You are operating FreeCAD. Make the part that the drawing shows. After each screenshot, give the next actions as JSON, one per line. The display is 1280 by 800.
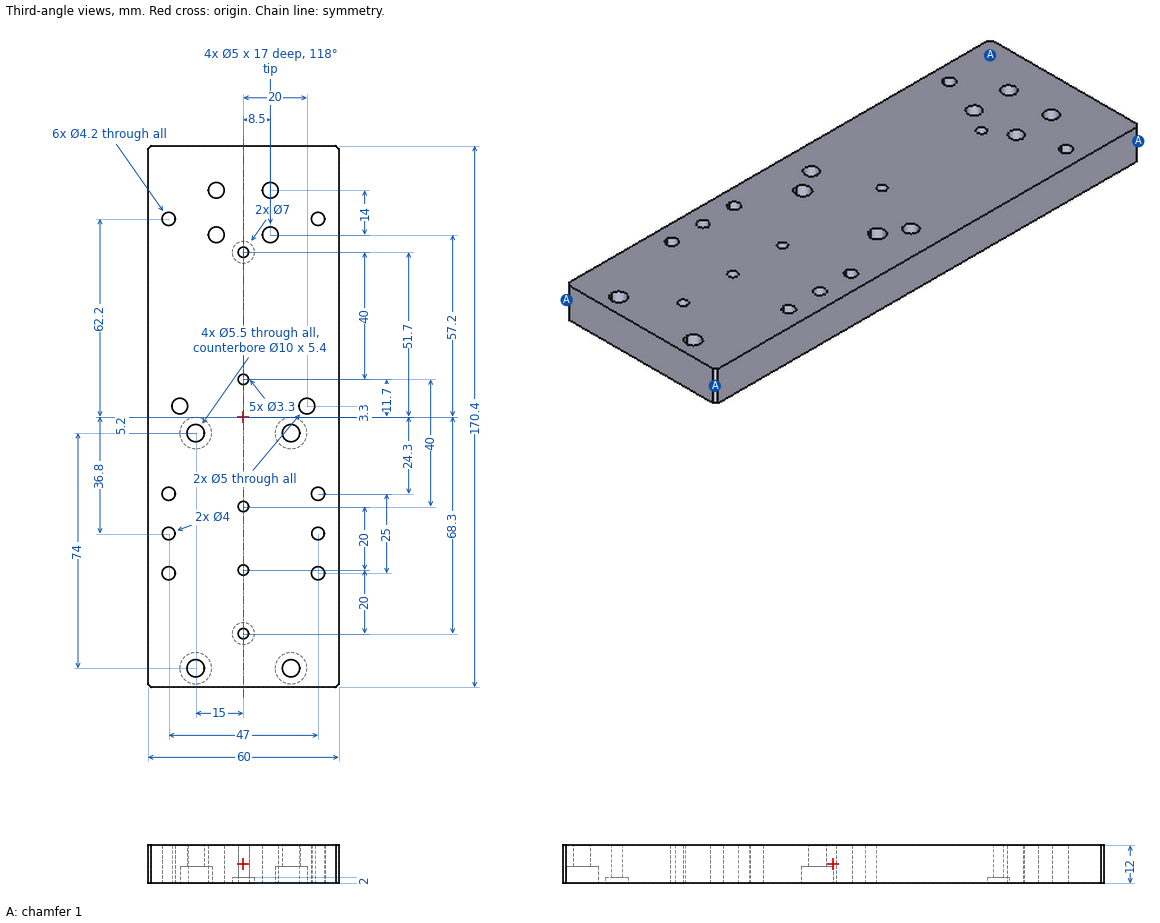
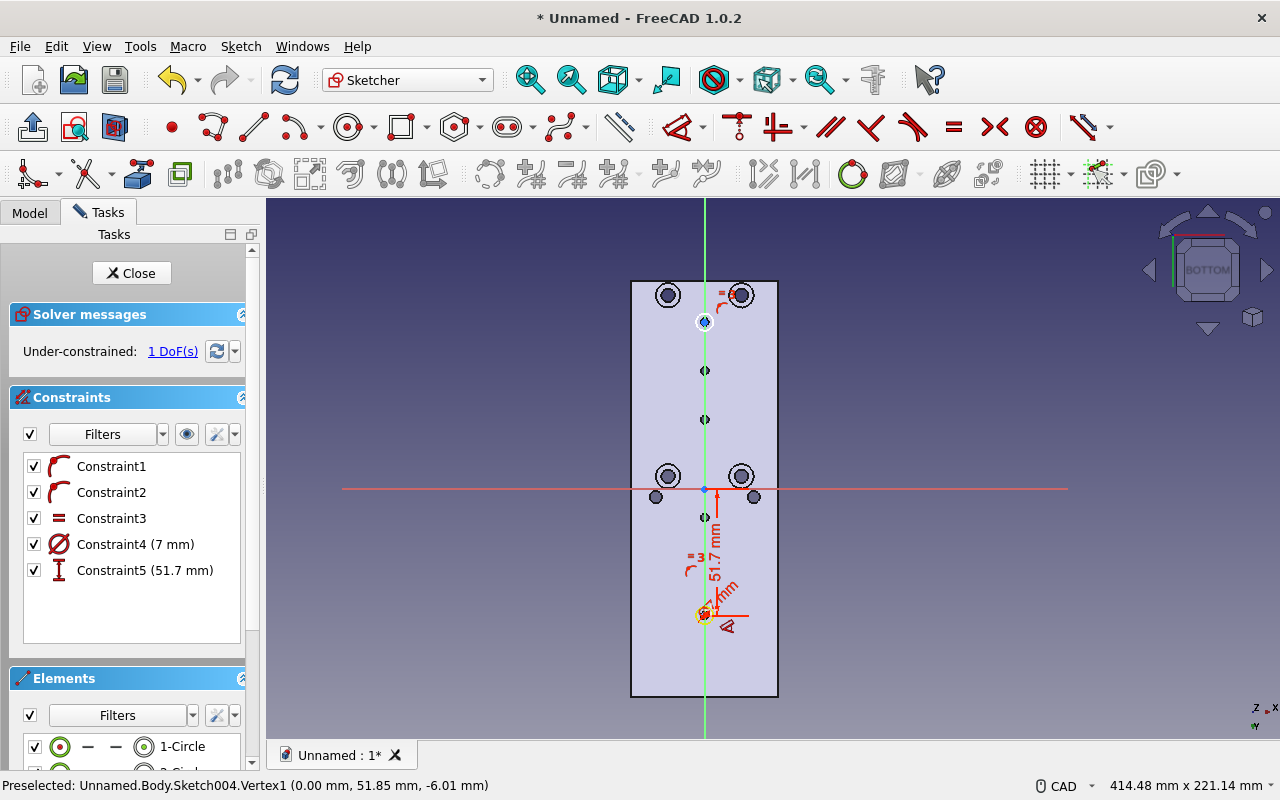
{"action": "left_click", "coordinate": [705, 322]}
{"action": "left_click", "coordinate": [739, 406]}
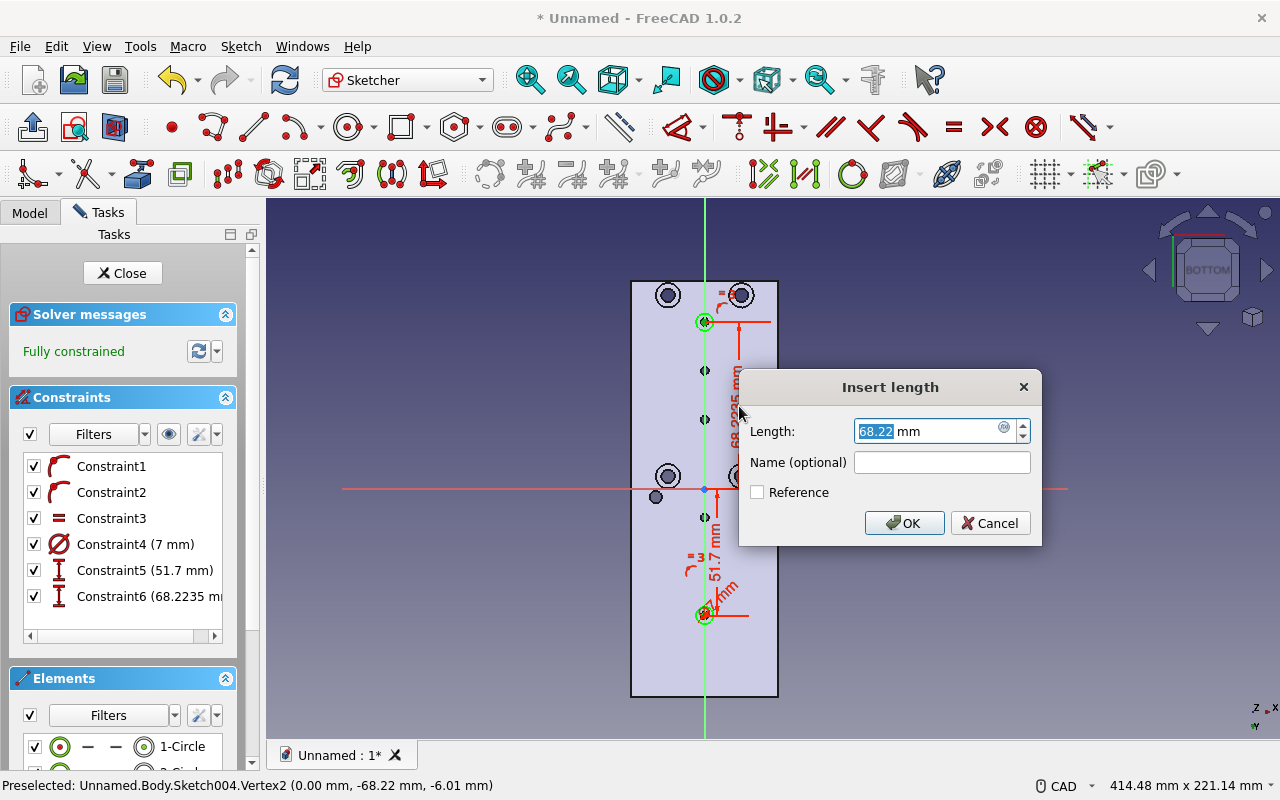
{"action": "type", "text": "68.3"}
{"action": "key", "text": "Return"}
{"action": "key", "text": "Escape"}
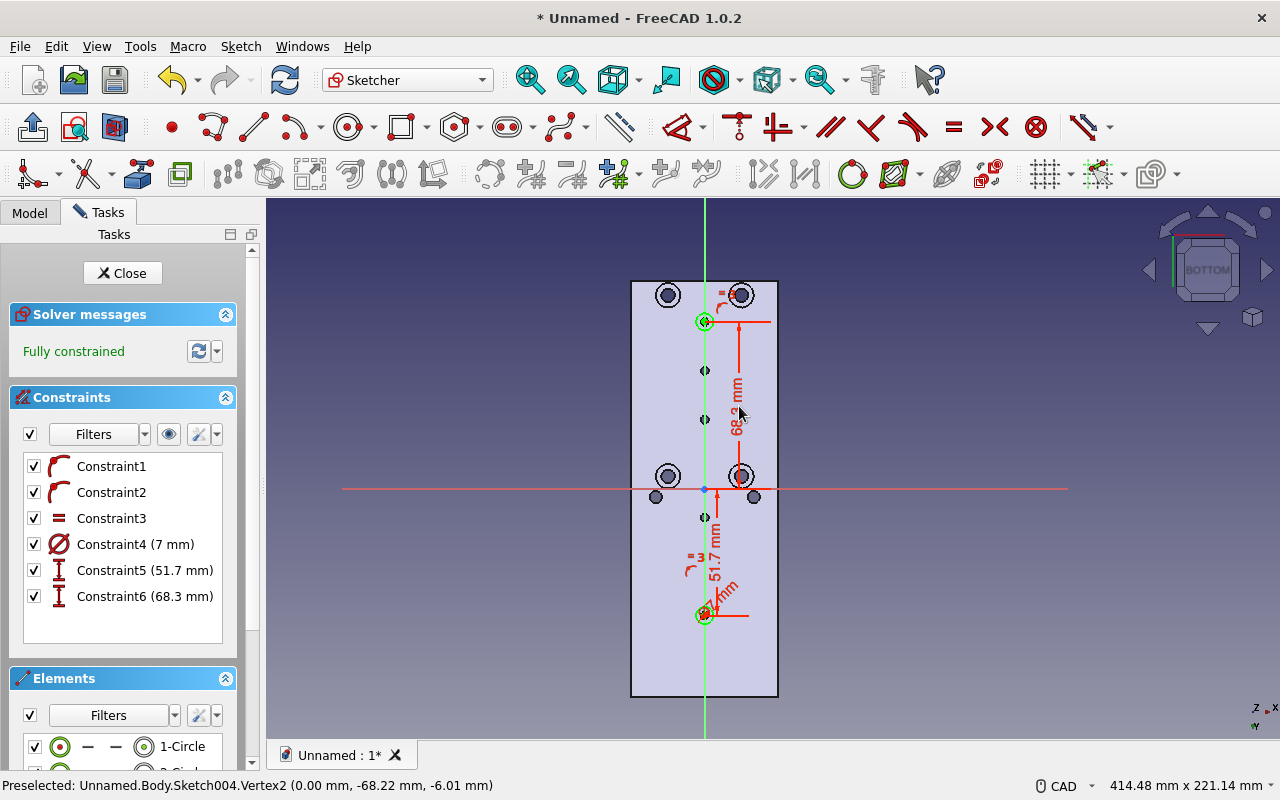
{"action": "left_click", "coordinate": [123, 273]}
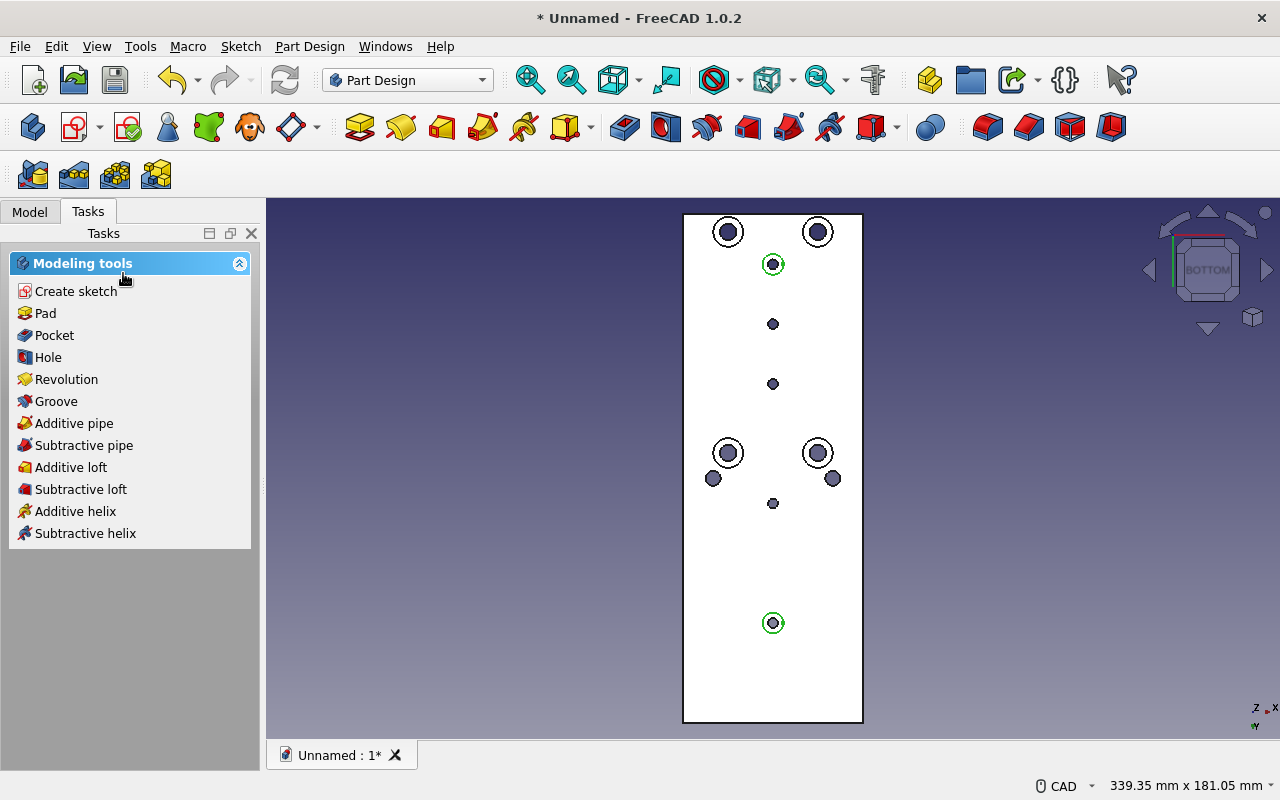
{"action": "left_click", "coordinate": [625, 128]}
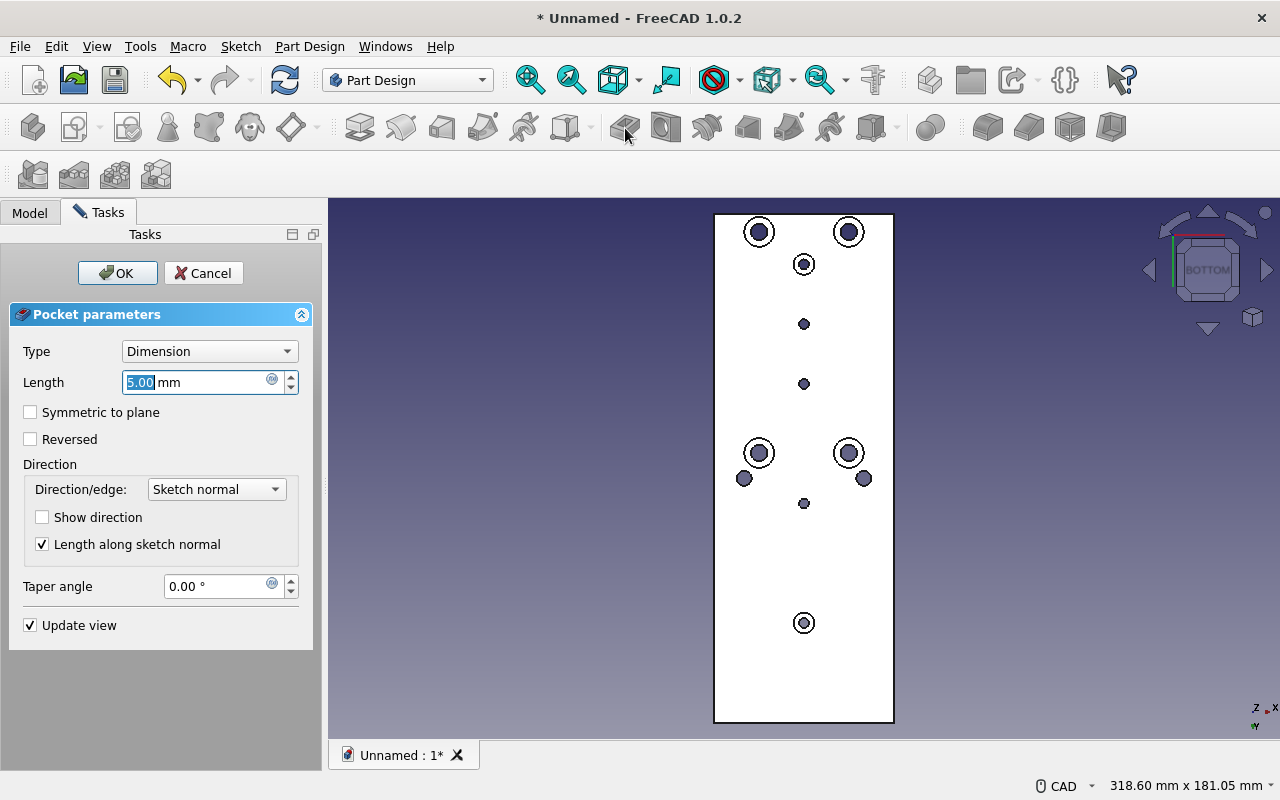
{"action": "type", "text": "2"}
{"action": "key", "text": "Tab"}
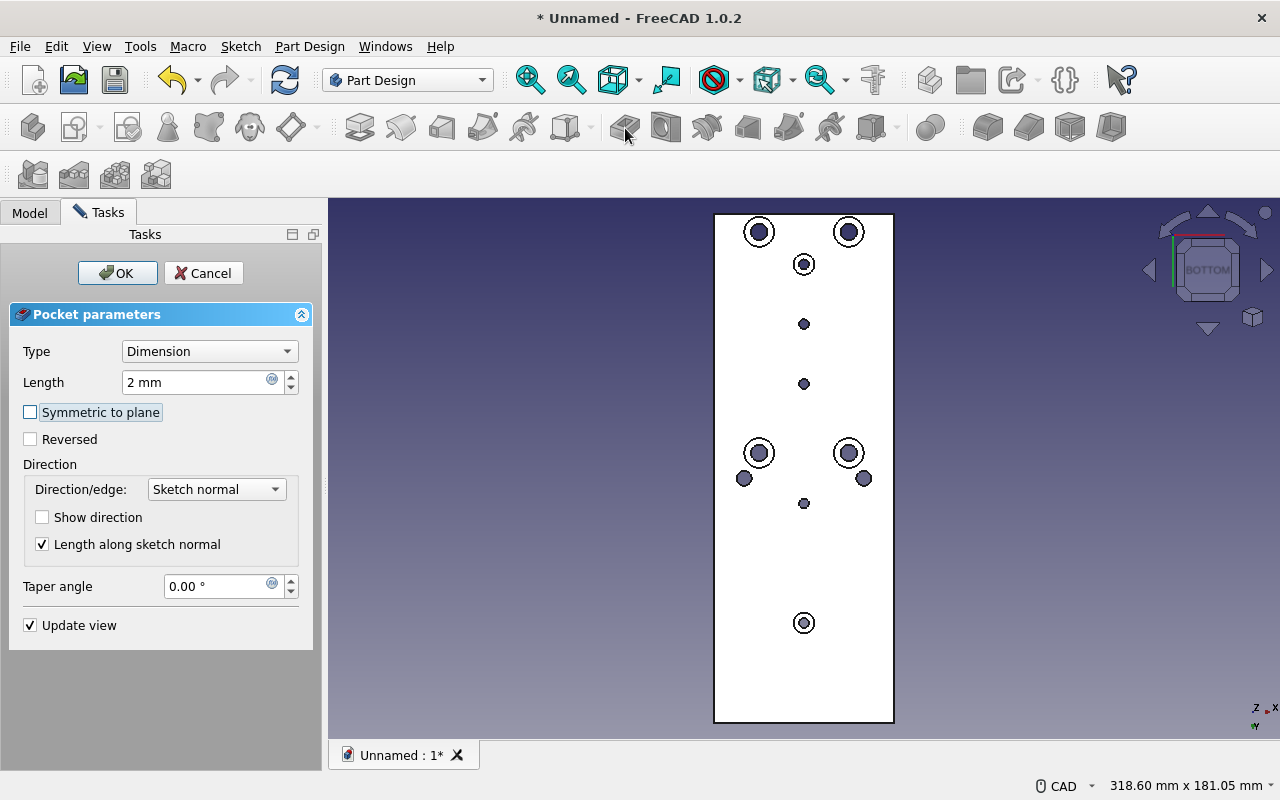
{"action": "left_click", "coordinate": [118, 273]}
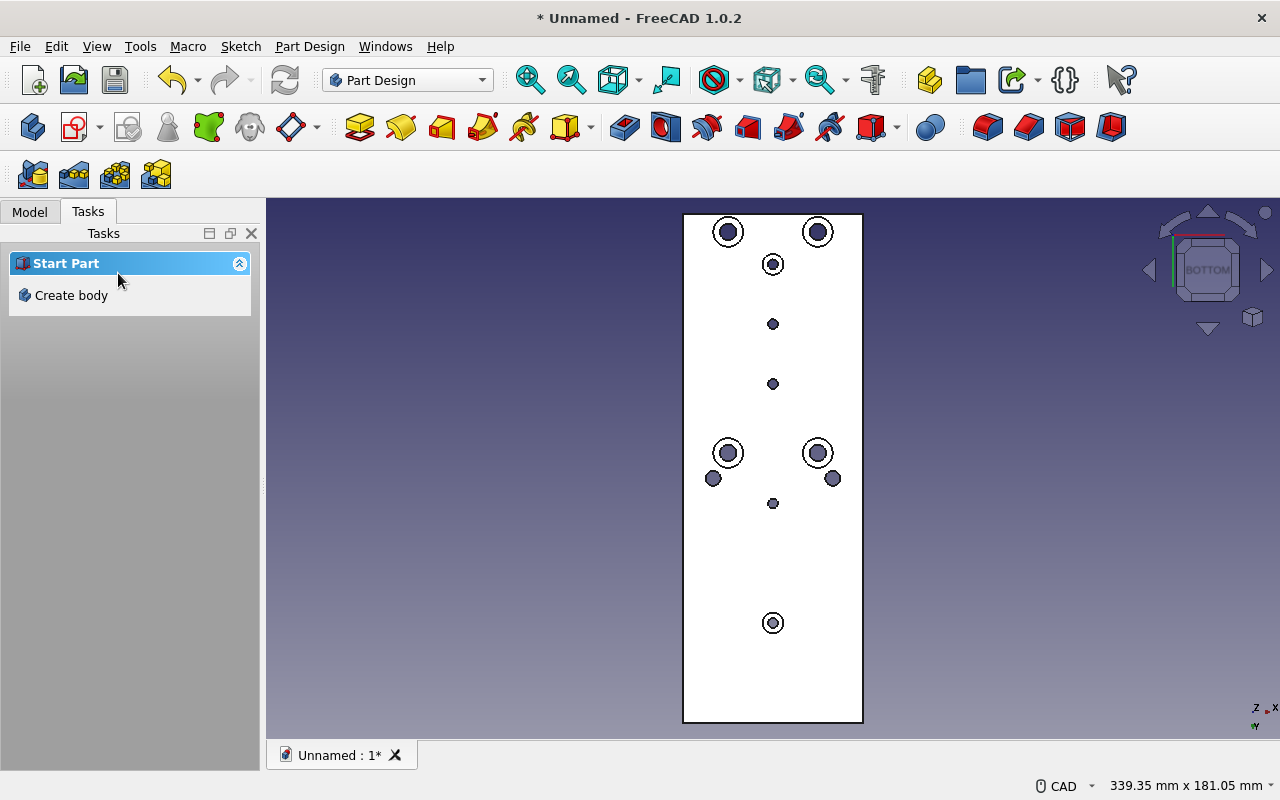
{"action": "key", "text": "0"}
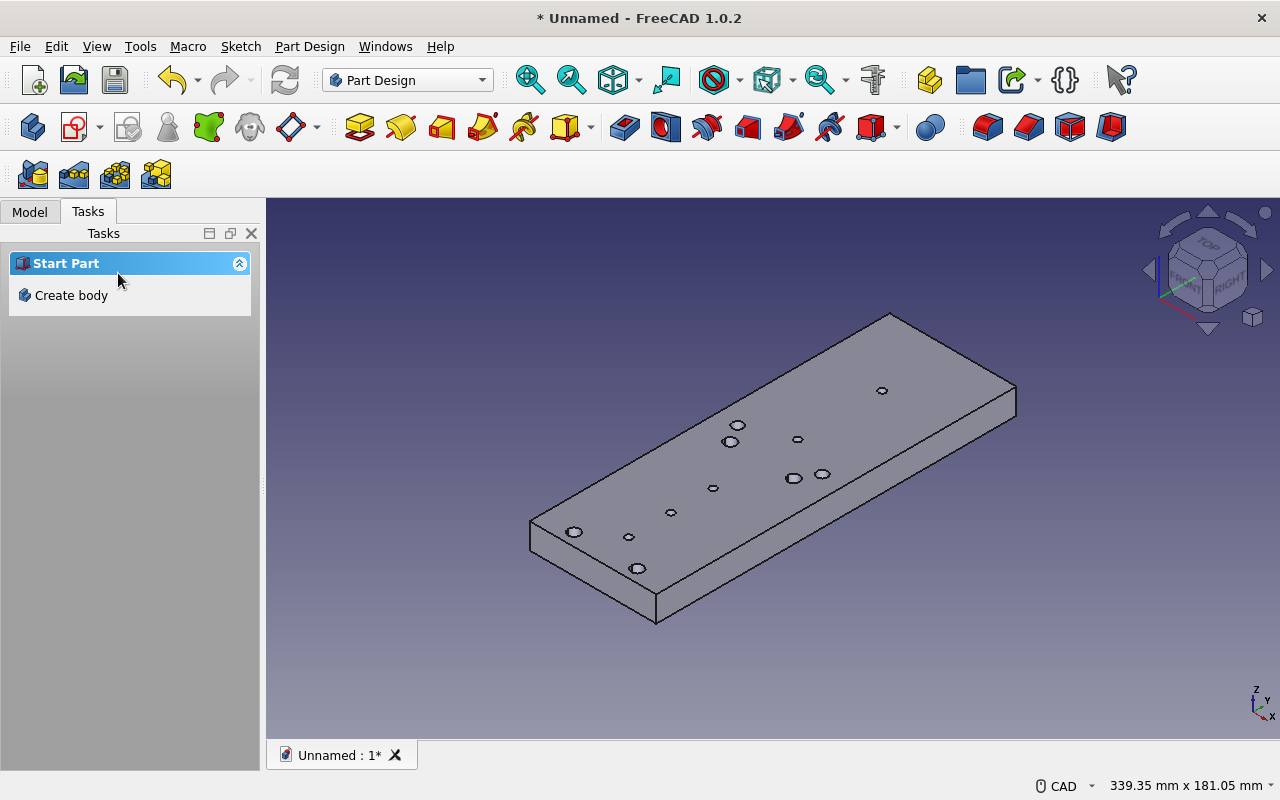
{"action": "left_click", "coordinate": [806, 413]}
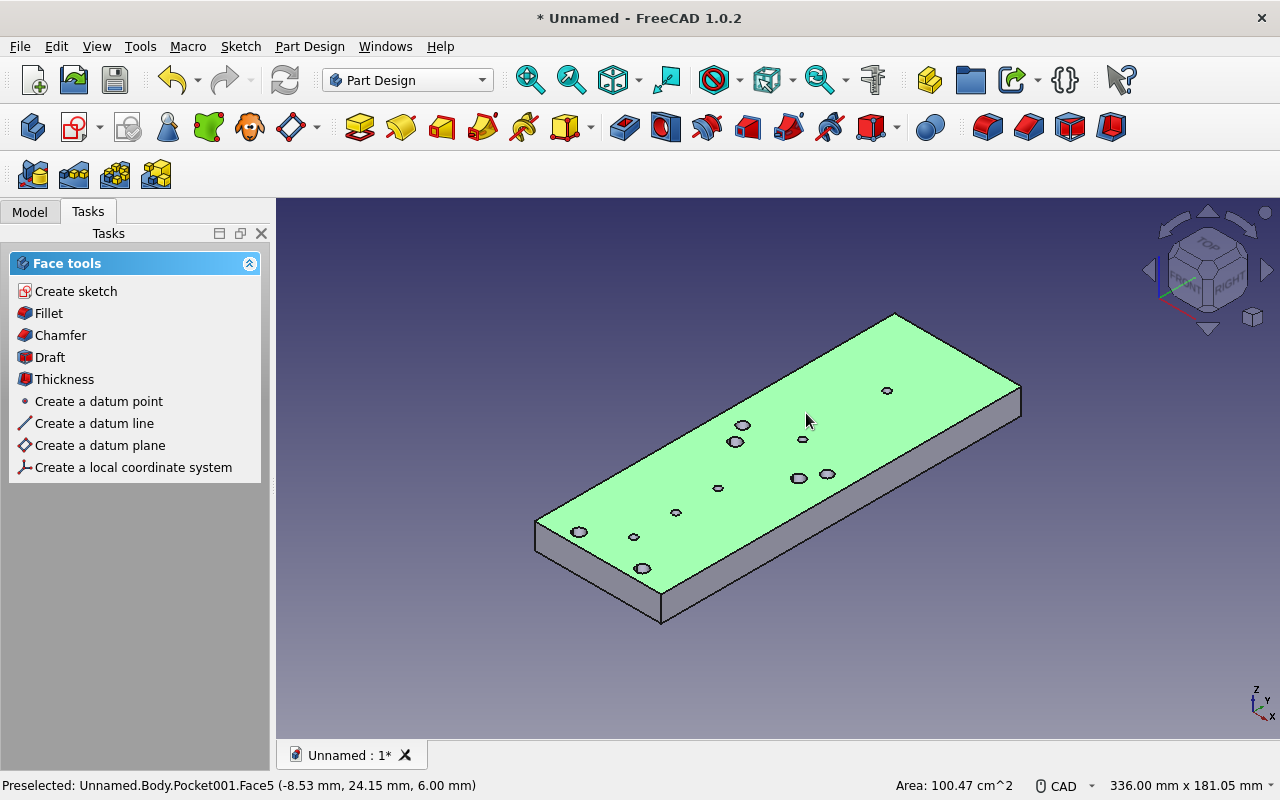
{"action": "left_click", "coordinate": [74, 128]}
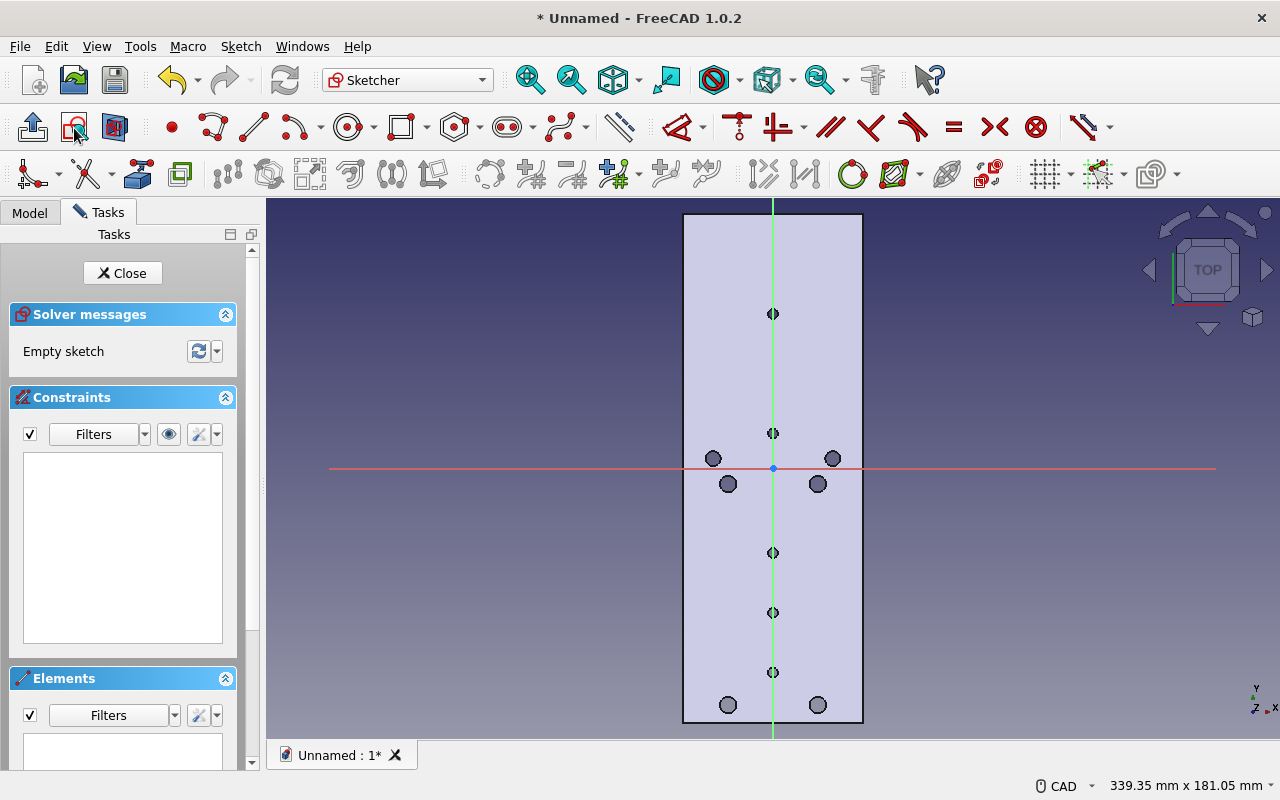
{"action": "scroll", "coordinate": [787, 239], "scroll_direction": "up", "scroll_amount": 9}